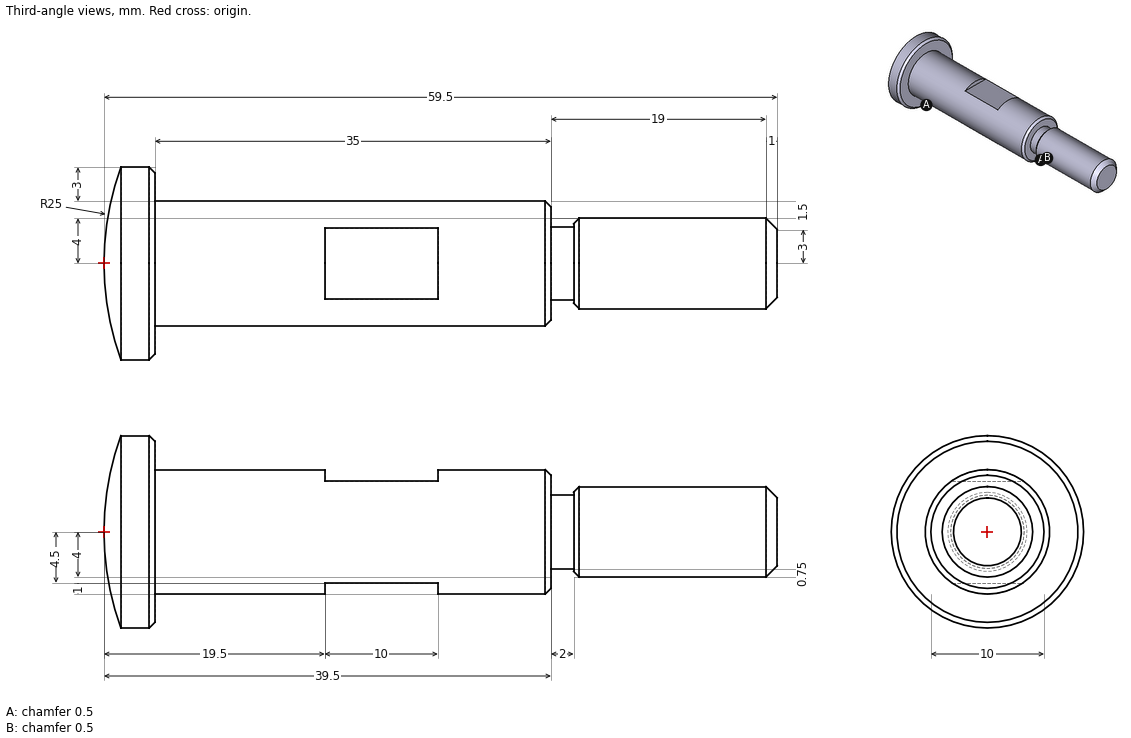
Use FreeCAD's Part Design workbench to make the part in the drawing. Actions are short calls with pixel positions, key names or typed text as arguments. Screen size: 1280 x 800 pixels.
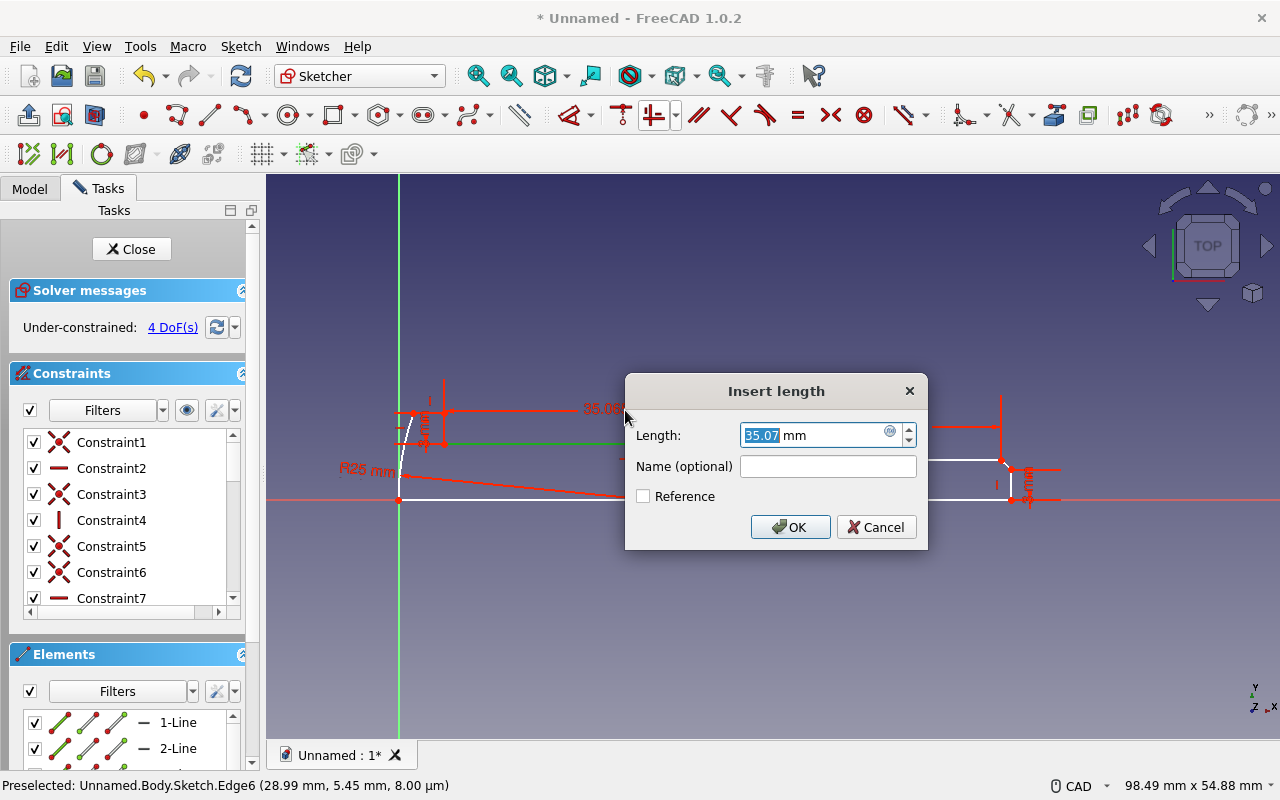
text(35)
key(Return)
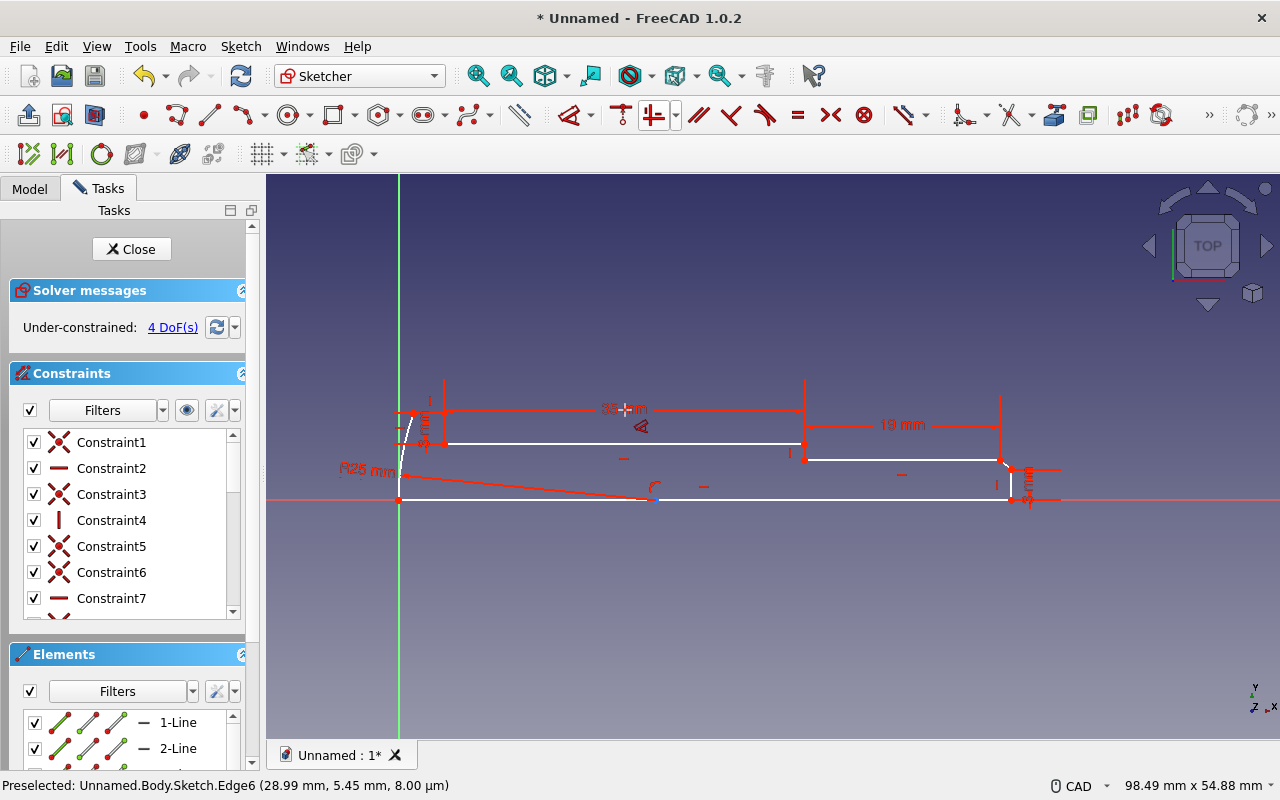
click(1000, 460)
click(1106, 480)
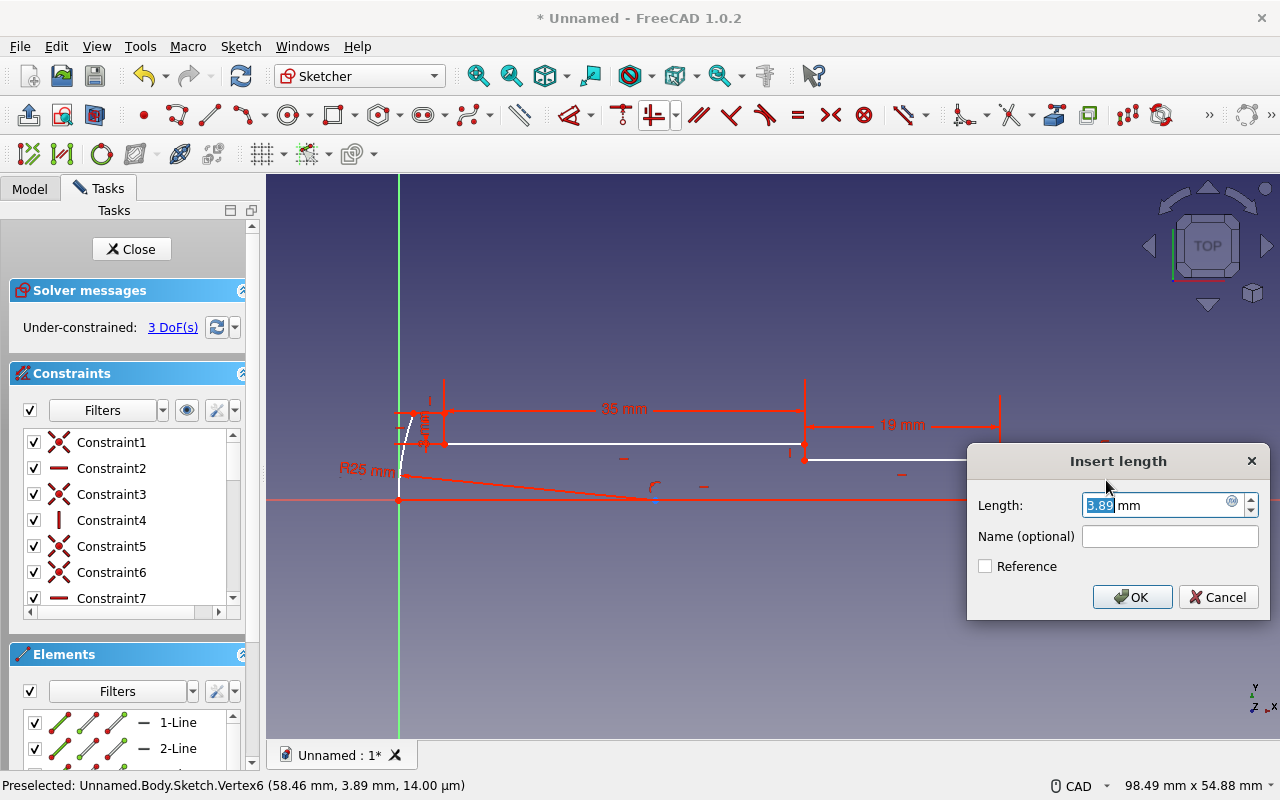
text(4)
key(Return)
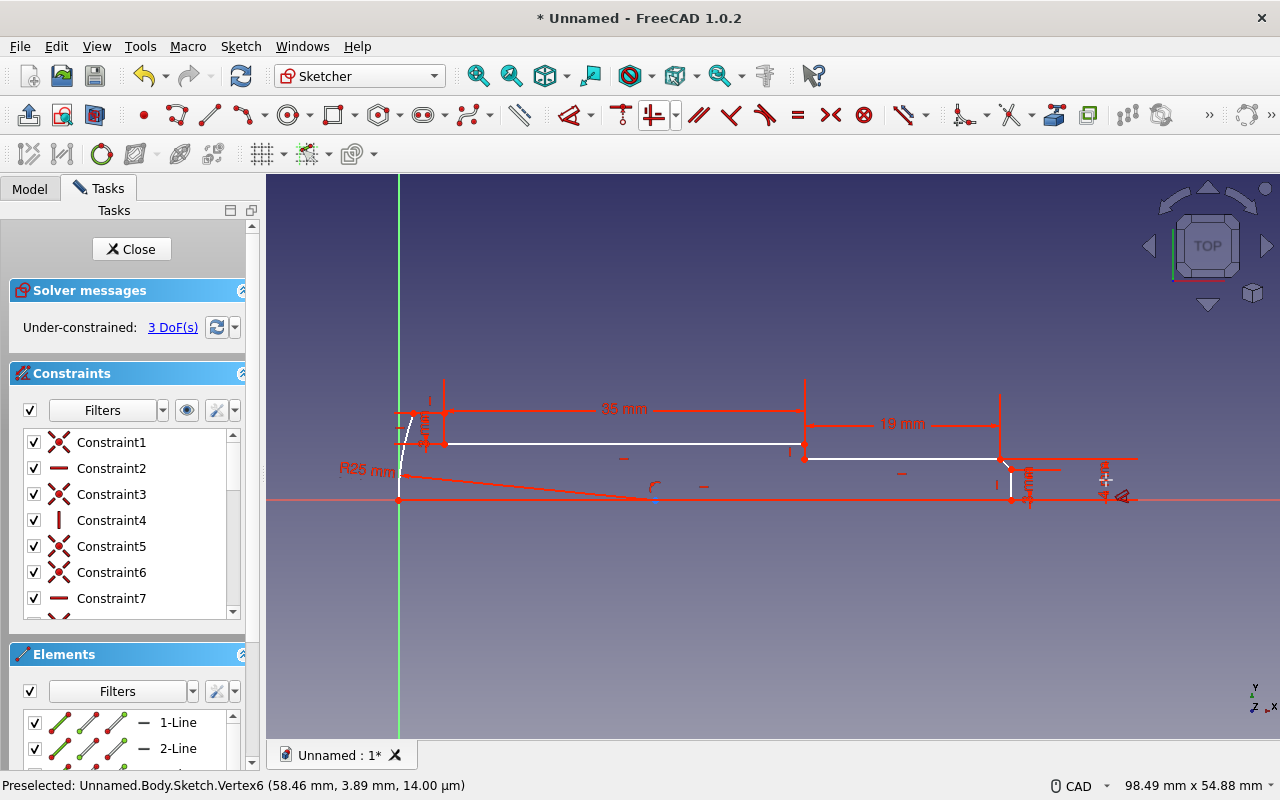
scroll(1006, 464, up, 7)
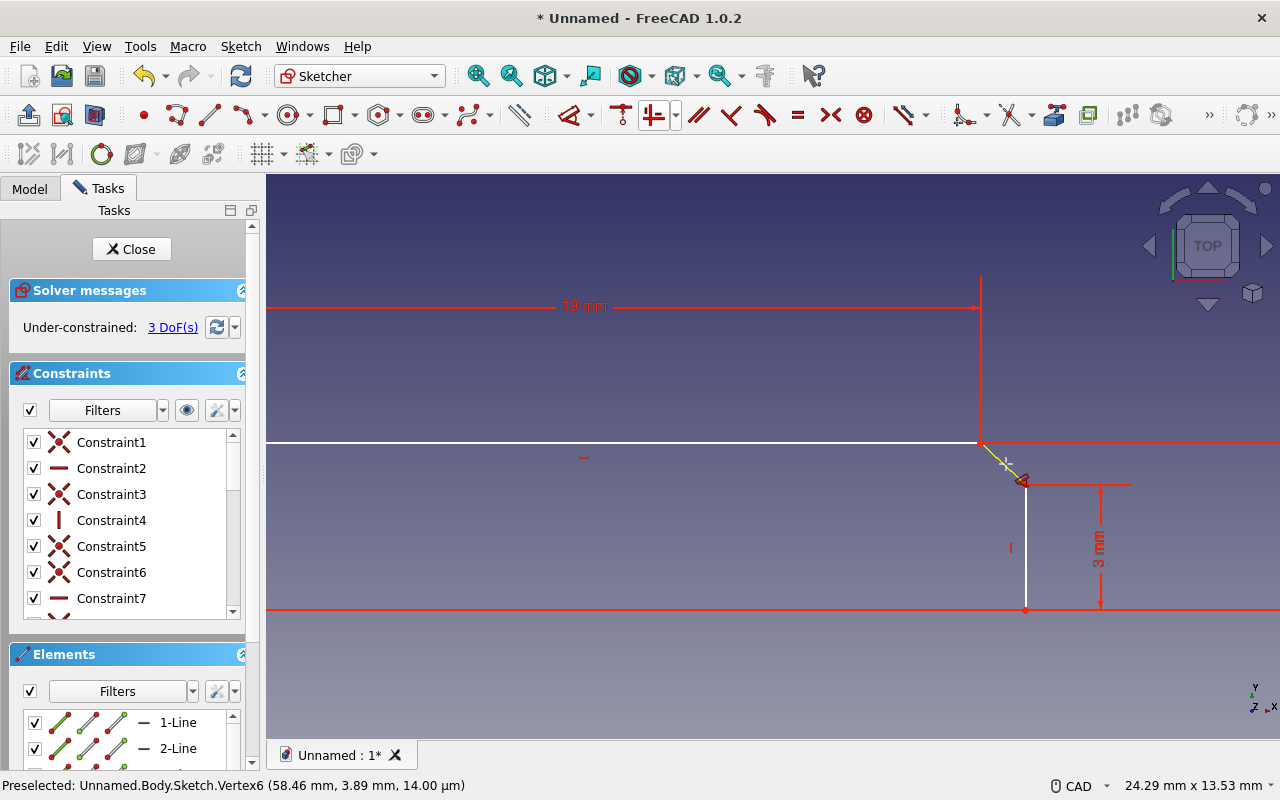
click(1003, 464)
click(1003, 519)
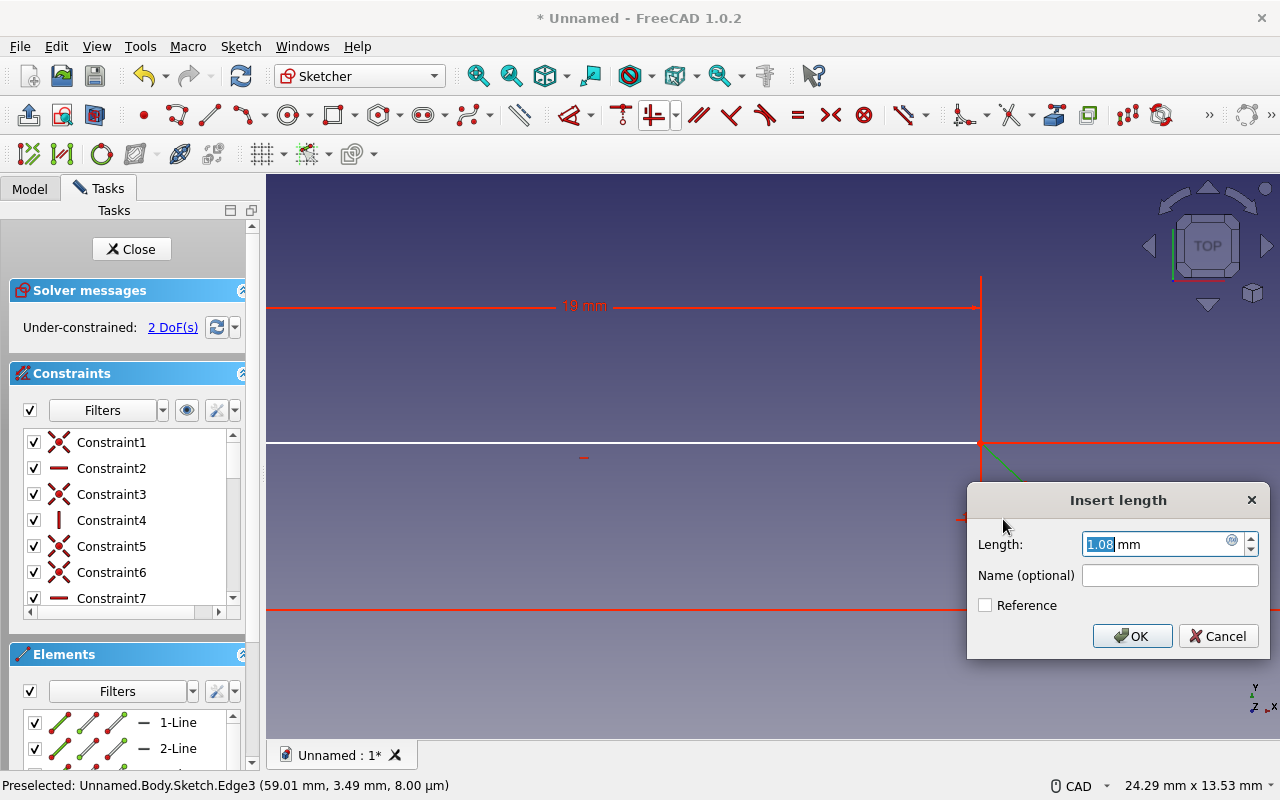
text(1)
key(Return)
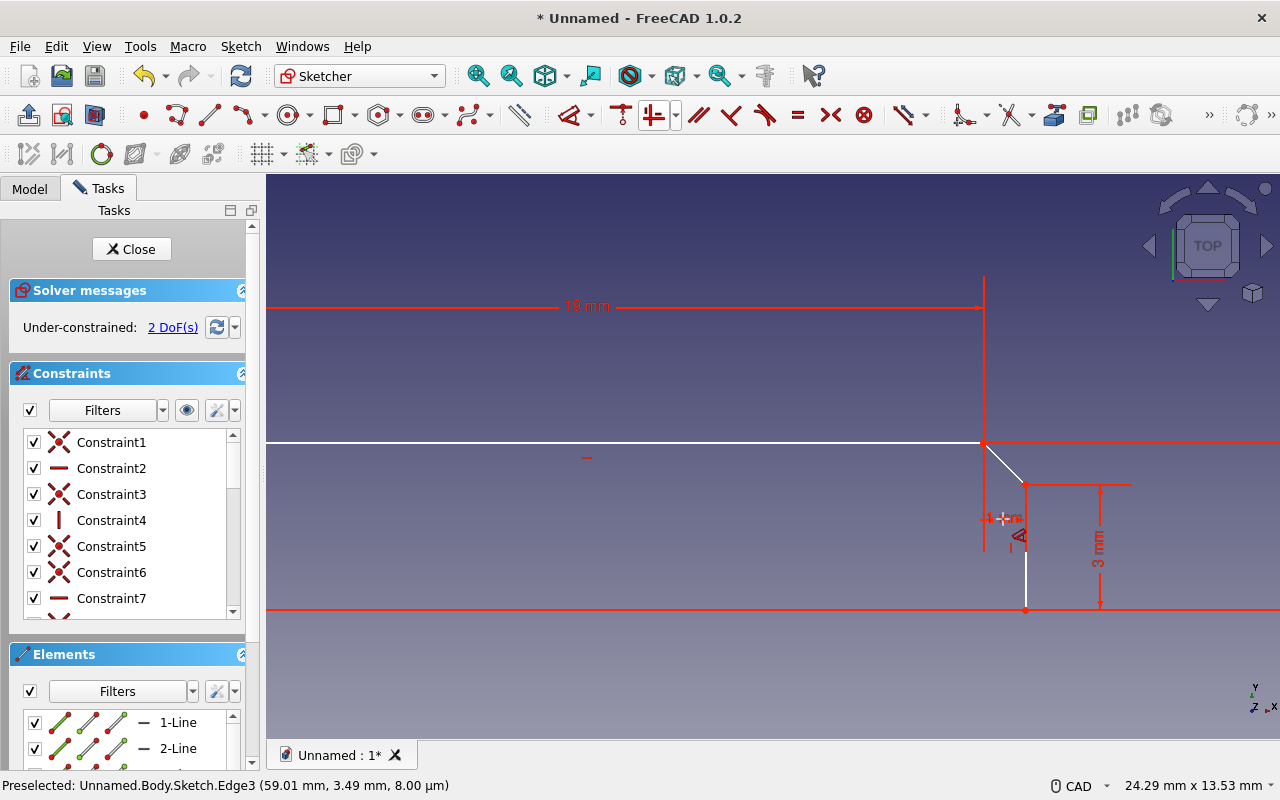
scroll(1006, 464, down, 7)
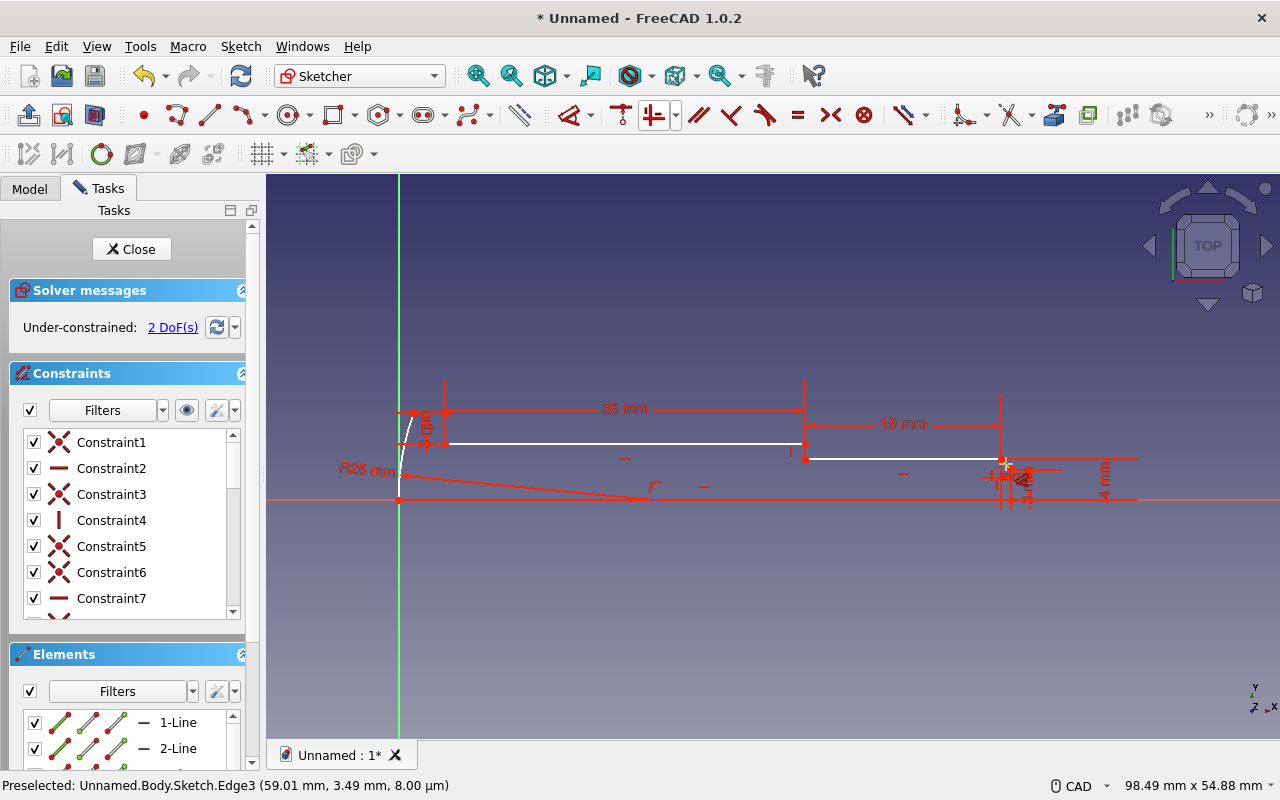
scroll(805, 455, up, 6)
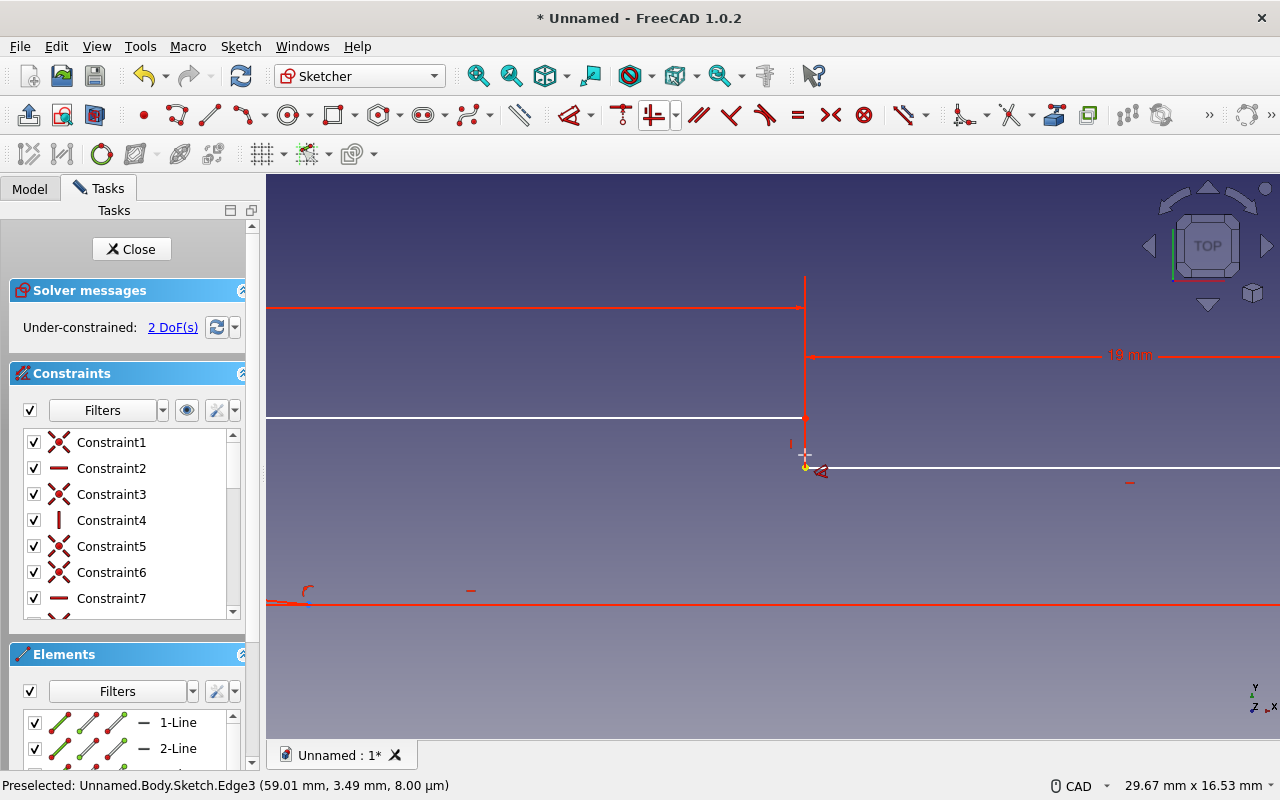
click(805, 453)
click(839, 443)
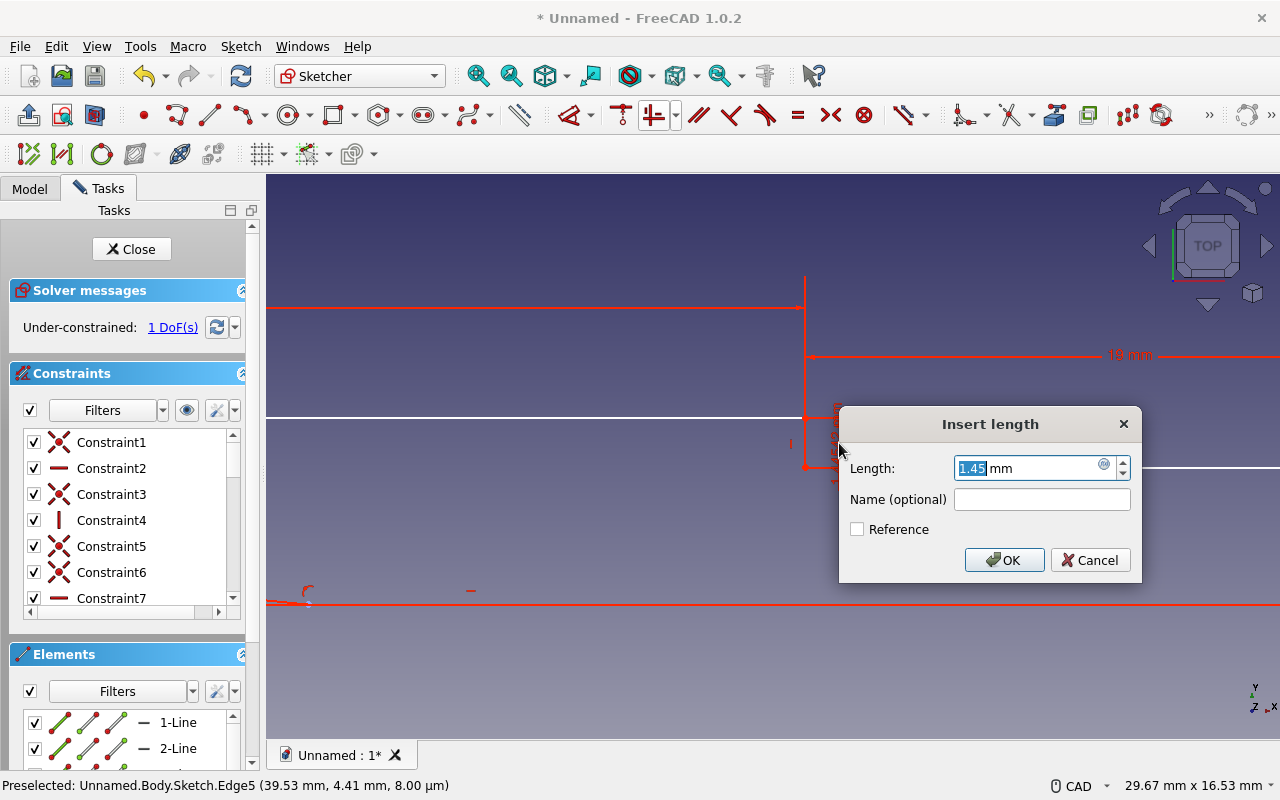
text(1.5)
key(Return)